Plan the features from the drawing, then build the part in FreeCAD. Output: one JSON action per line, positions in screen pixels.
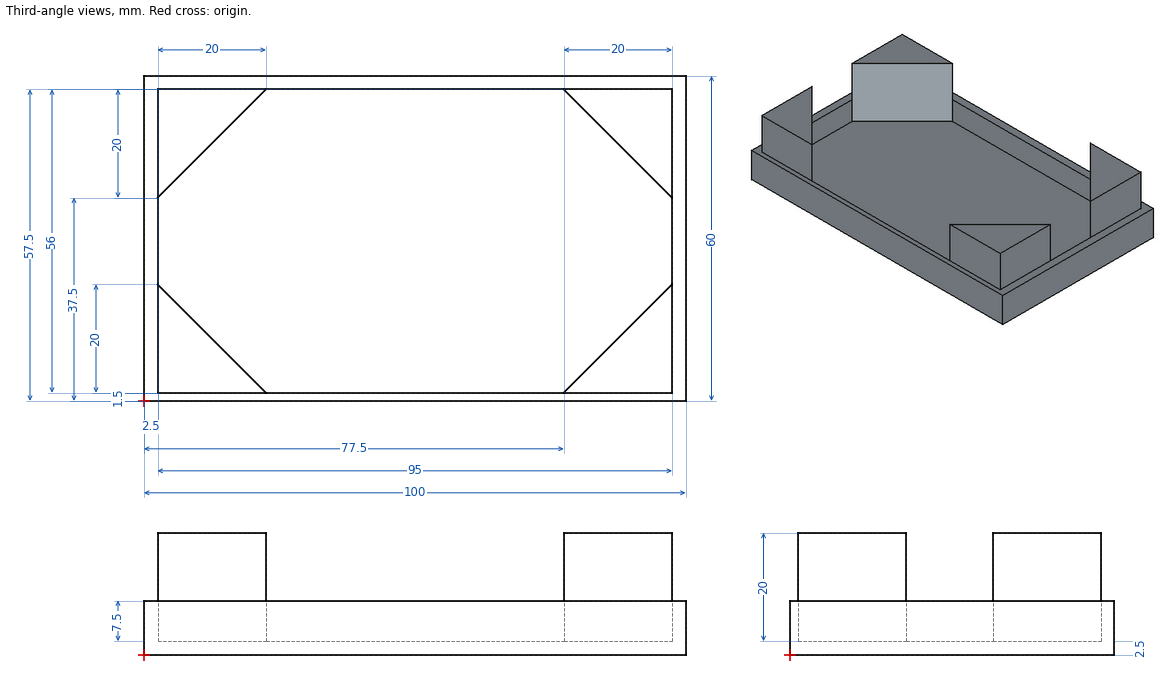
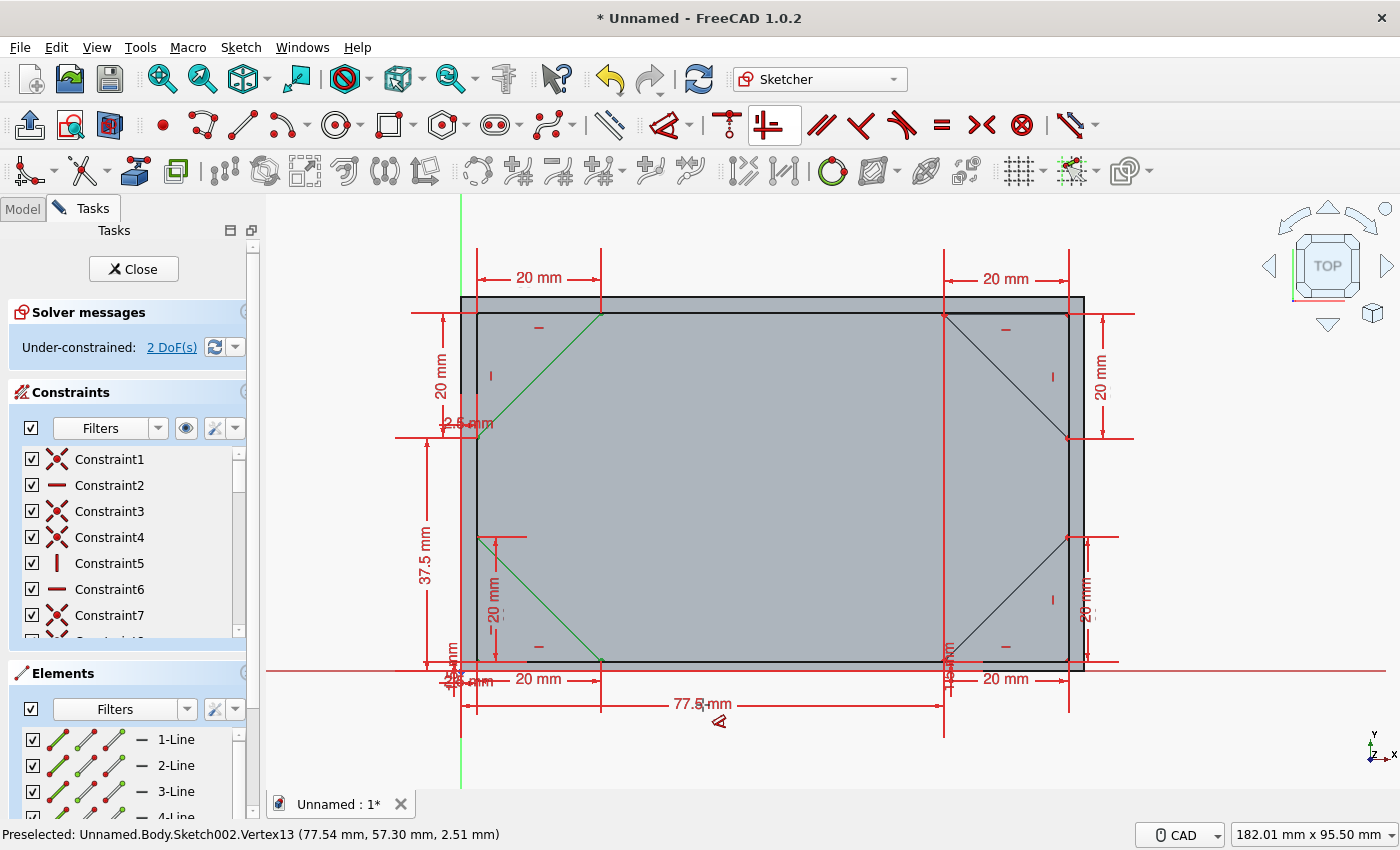
{"action": "left_click", "coordinate": [944, 314]}
{"action": "left_click", "coordinate": [427, 493]}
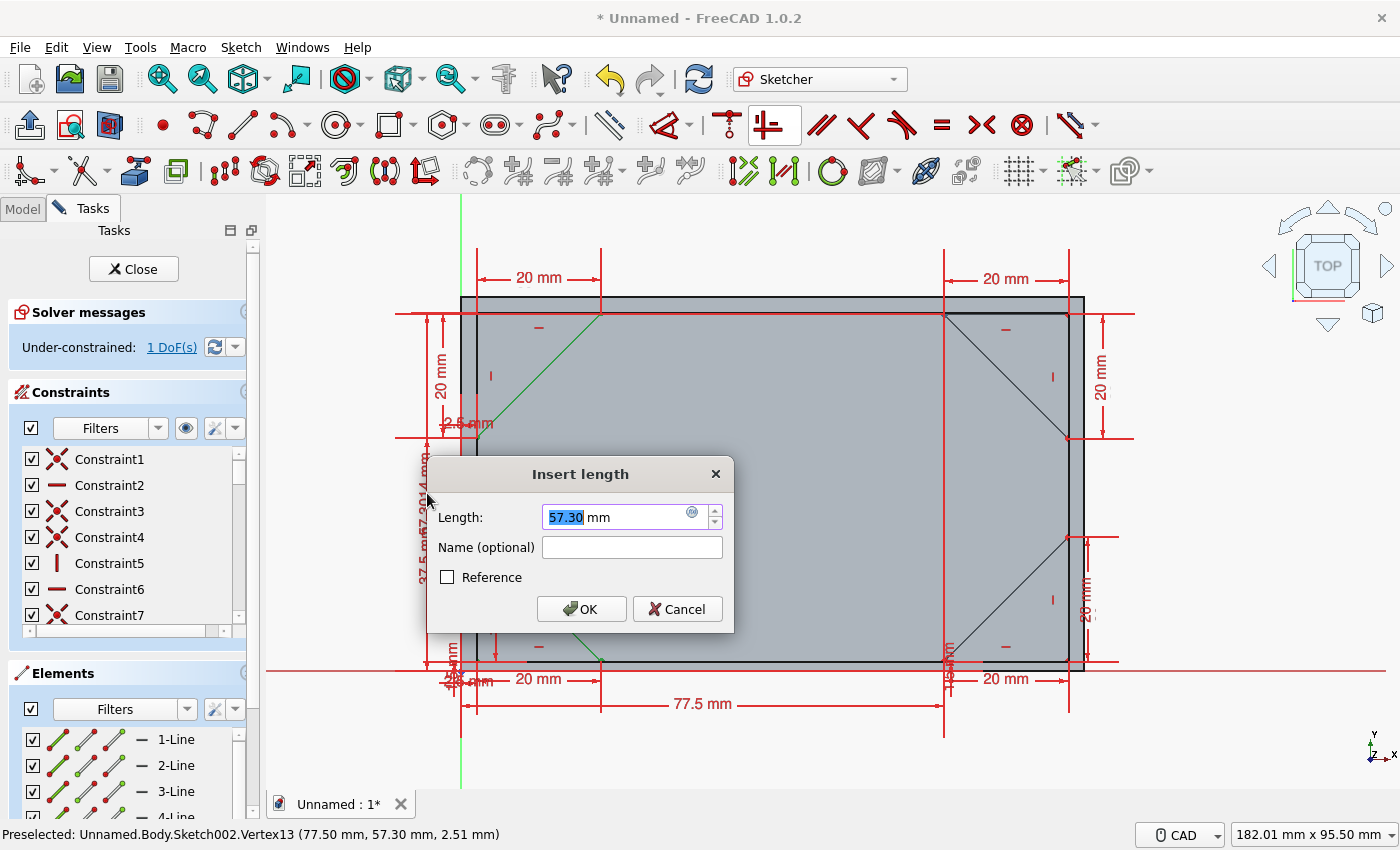
{"action": "type", "text": "57.5"}
{"action": "key", "text": "Return"}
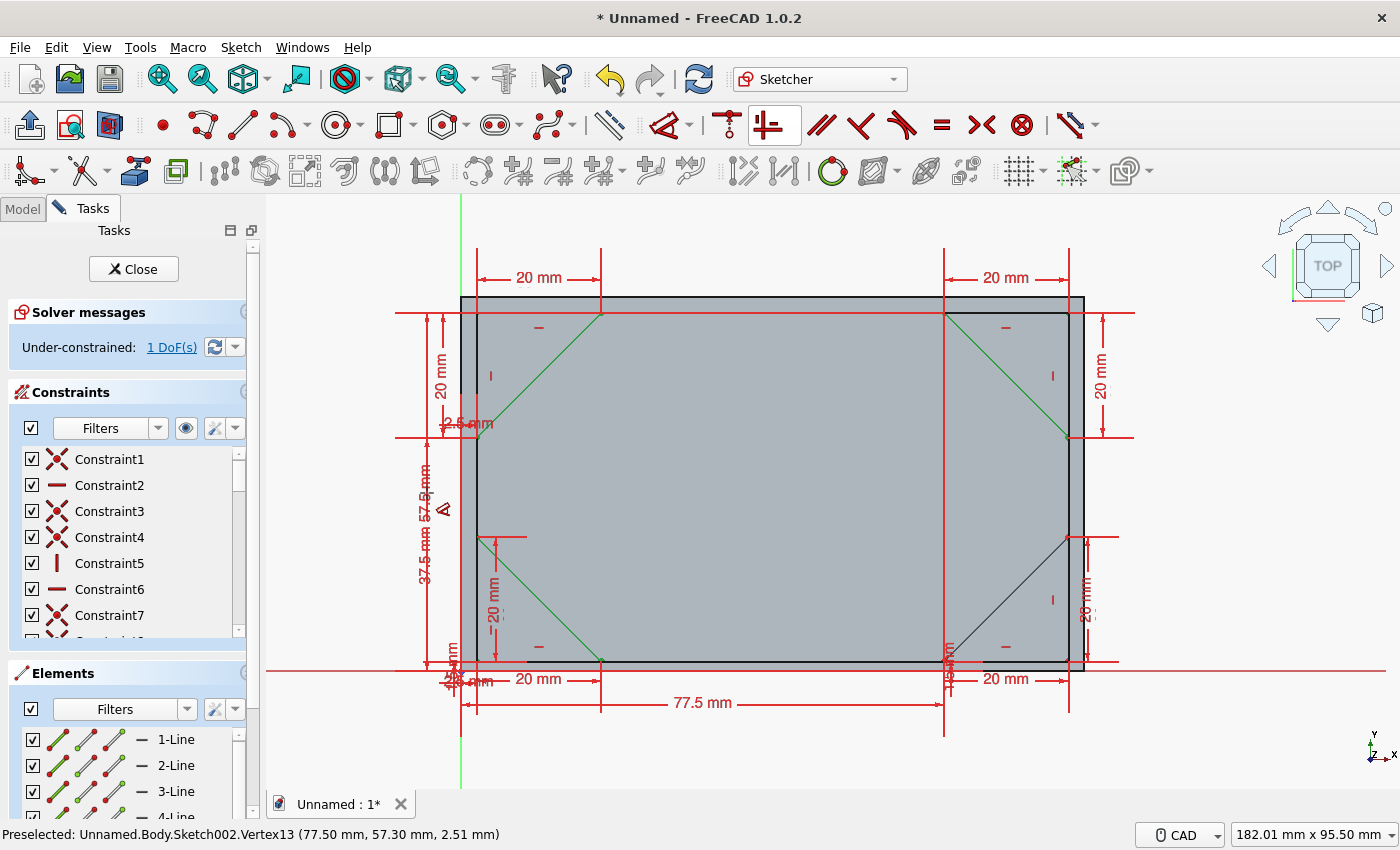
{"action": "left_click", "coordinate": [944, 662]}
{"action": "left_click", "coordinate": [592, 705]}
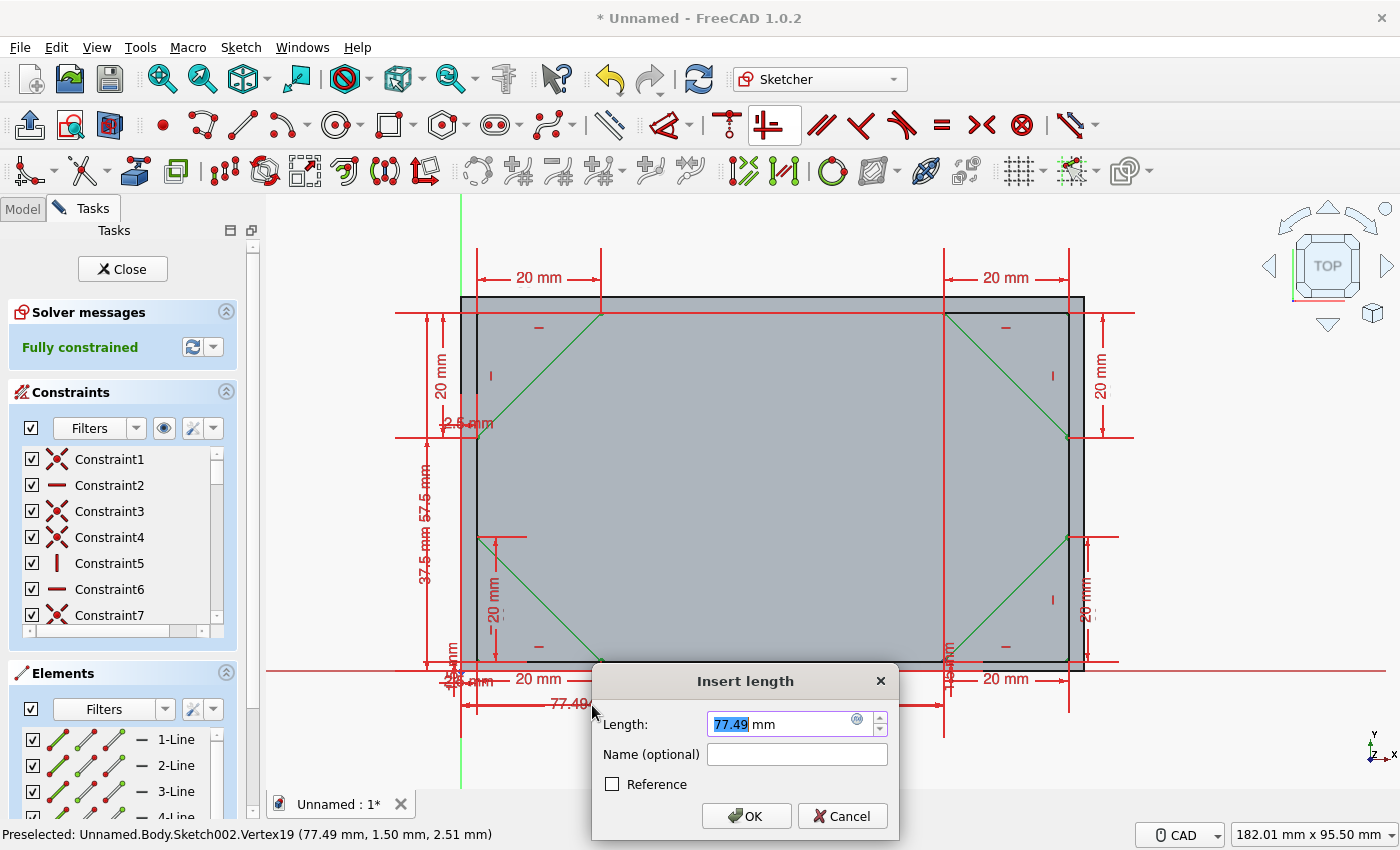
{"action": "type", "text": "77.5"}
{"action": "key", "text": "Return"}
{"action": "key", "text": "Escape"}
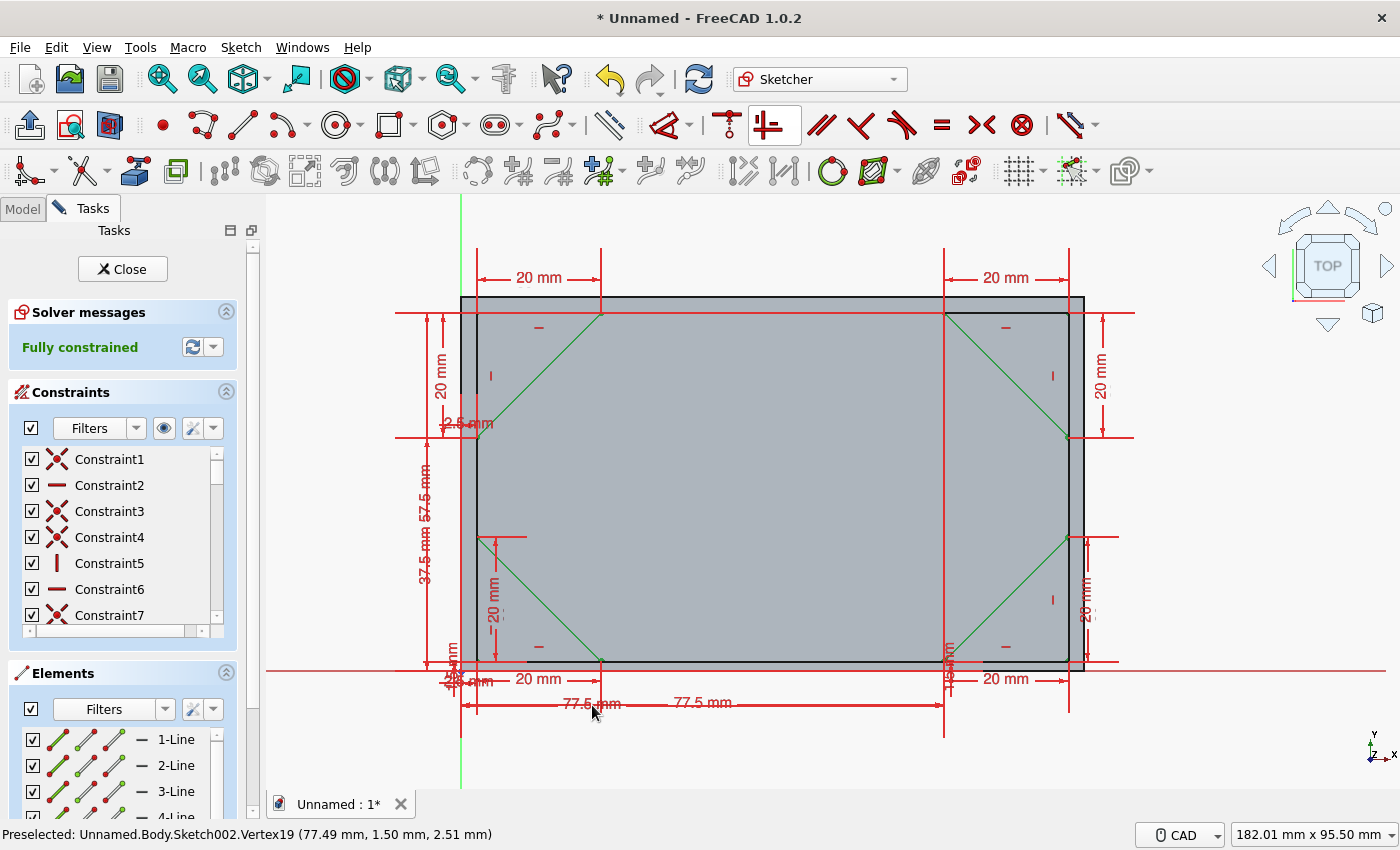
{"action": "left_click", "coordinate": [123, 269]}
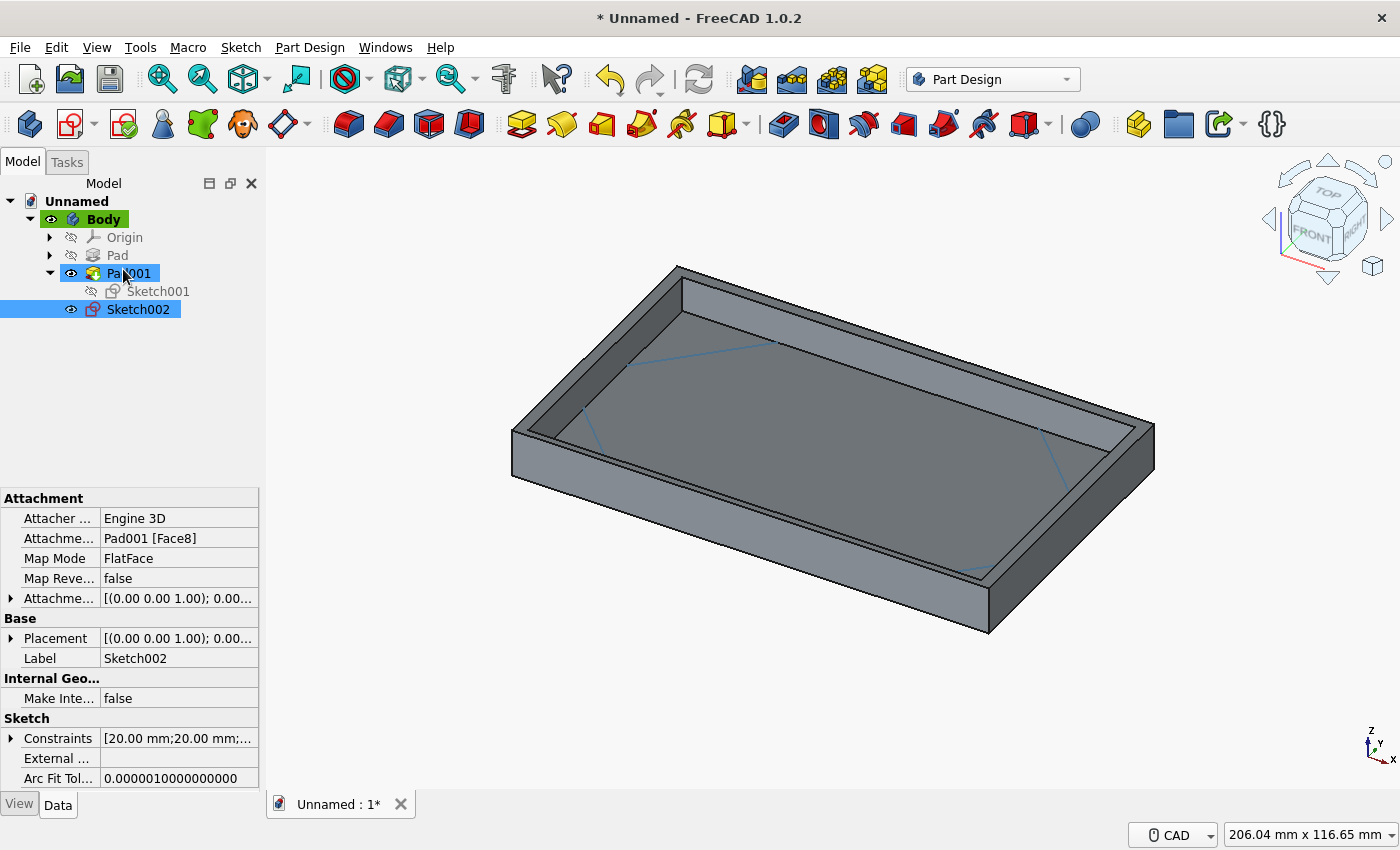
{"action": "left_click", "coordinate": [522, 124]}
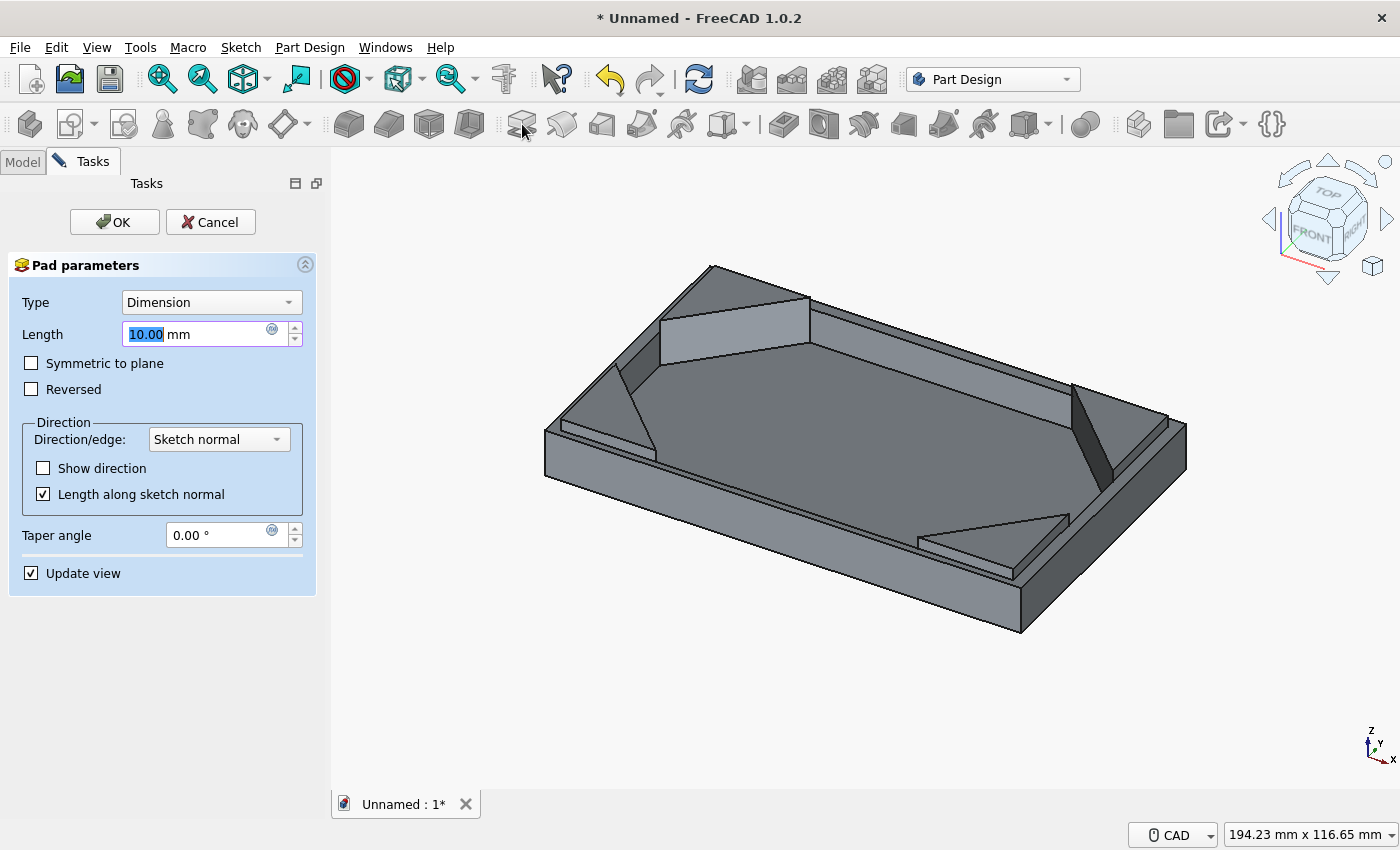
{"action": "type", "text": "20"}
{"action": "key", "text": "Tab"}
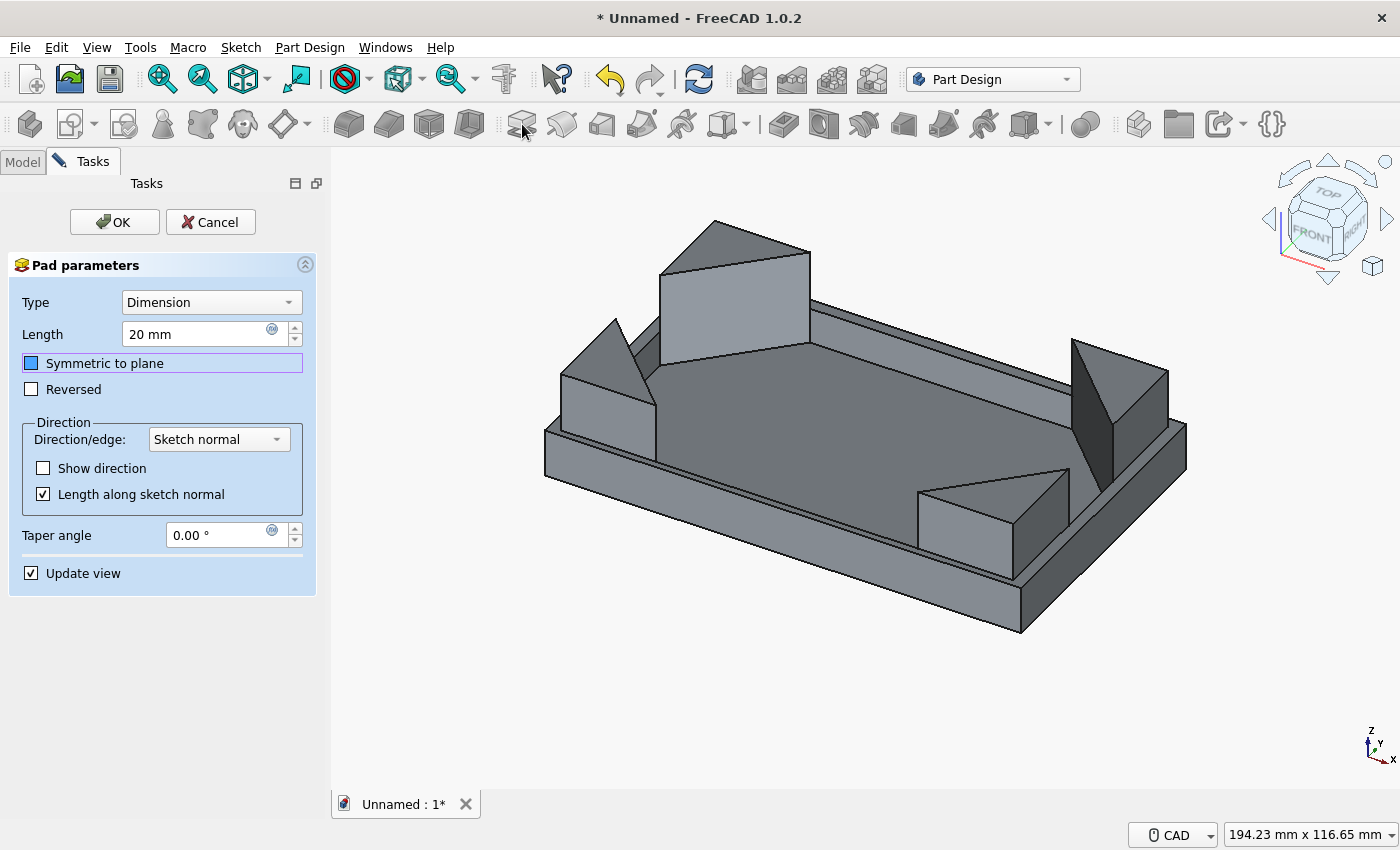
{"action": "left_click", "coordinate": [115, 222]}